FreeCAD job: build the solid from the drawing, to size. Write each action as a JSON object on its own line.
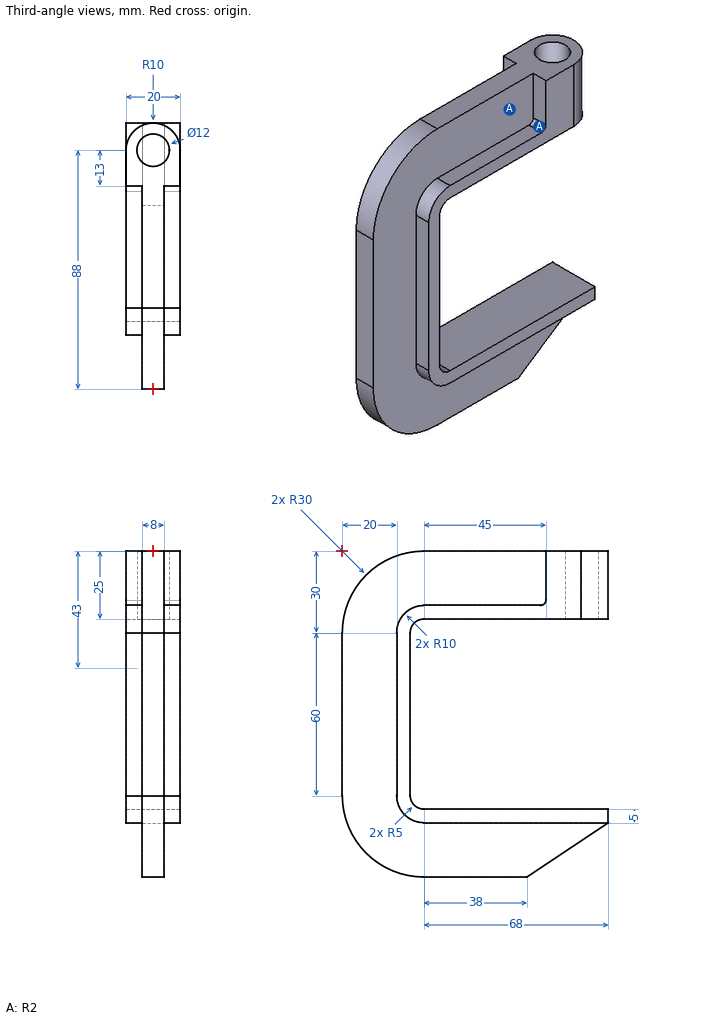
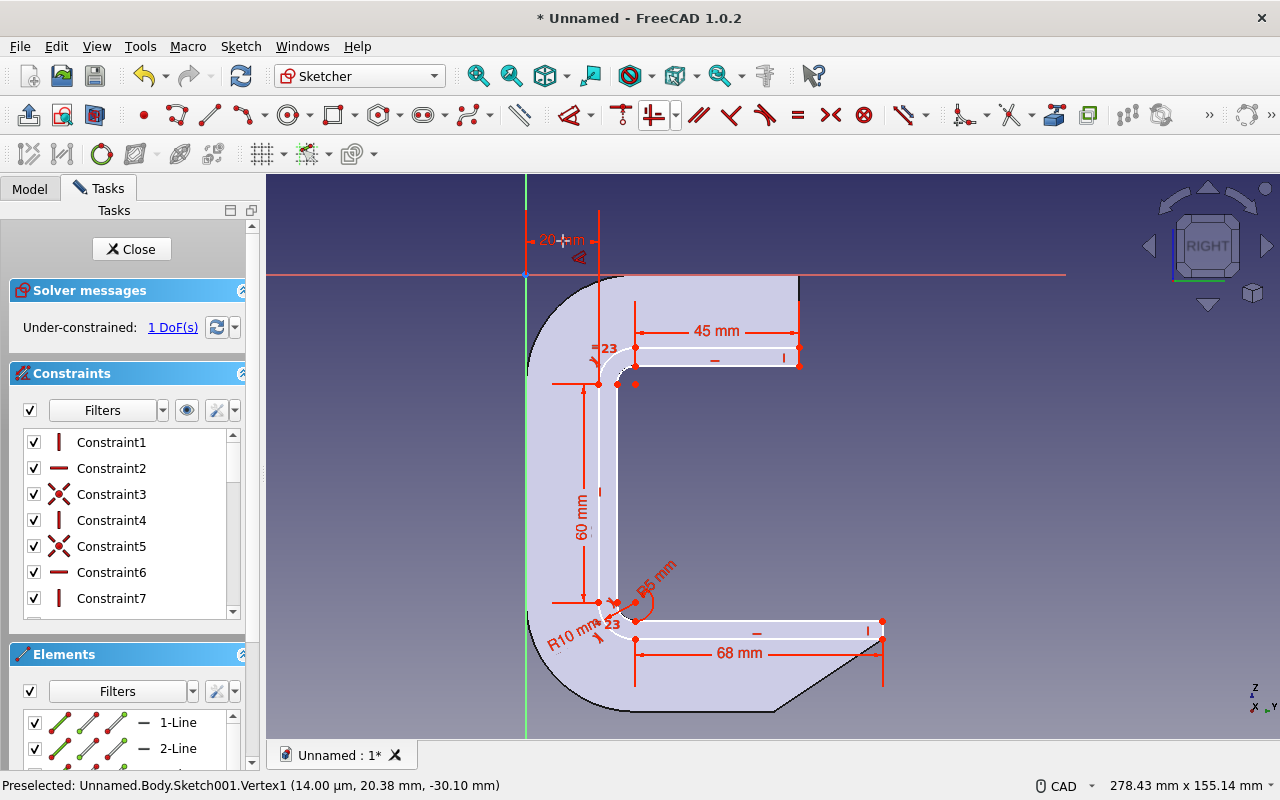
{"action": "left_click", "coordinate": [599, 384]}
{"action": "left_click", "coordinate": [492, 330]}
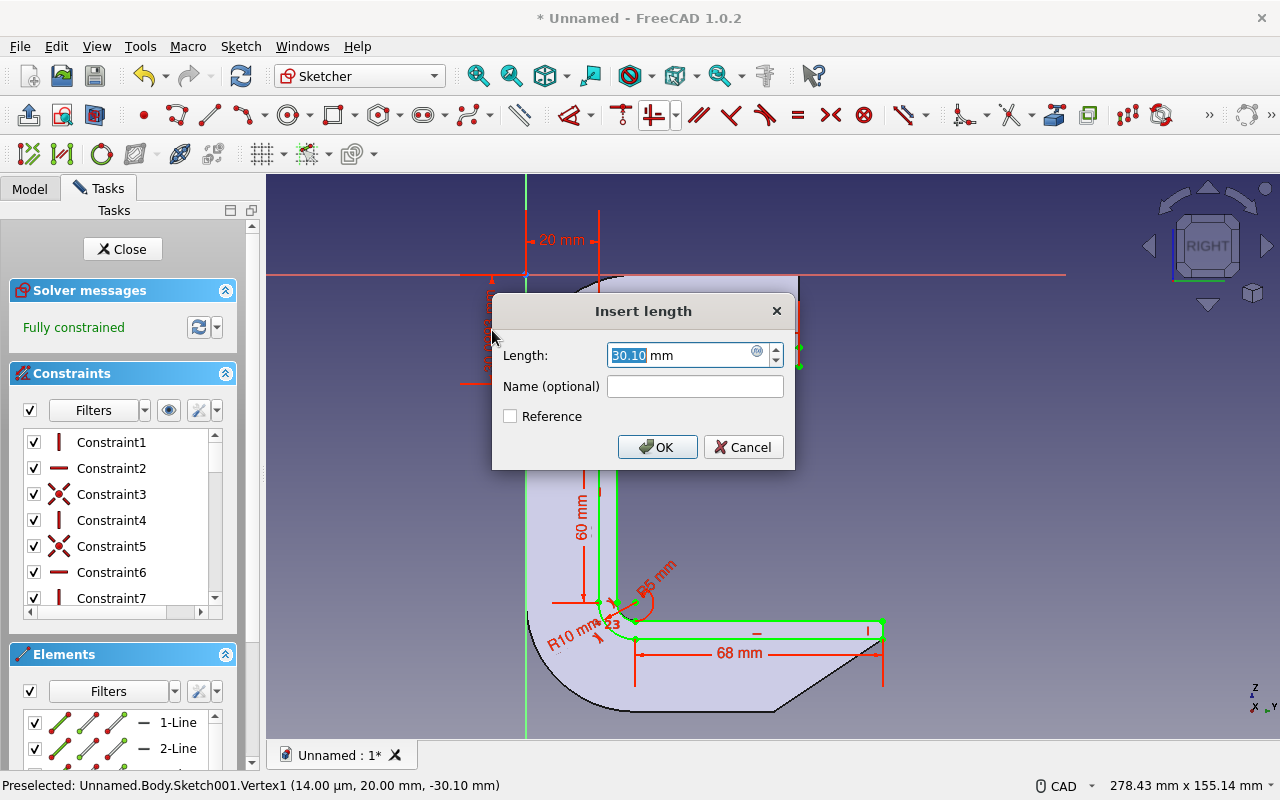
{"action": "type", "text": "30"}
{"action": "key", "text": "Return"}
{"action": "key", "text": "Escape"}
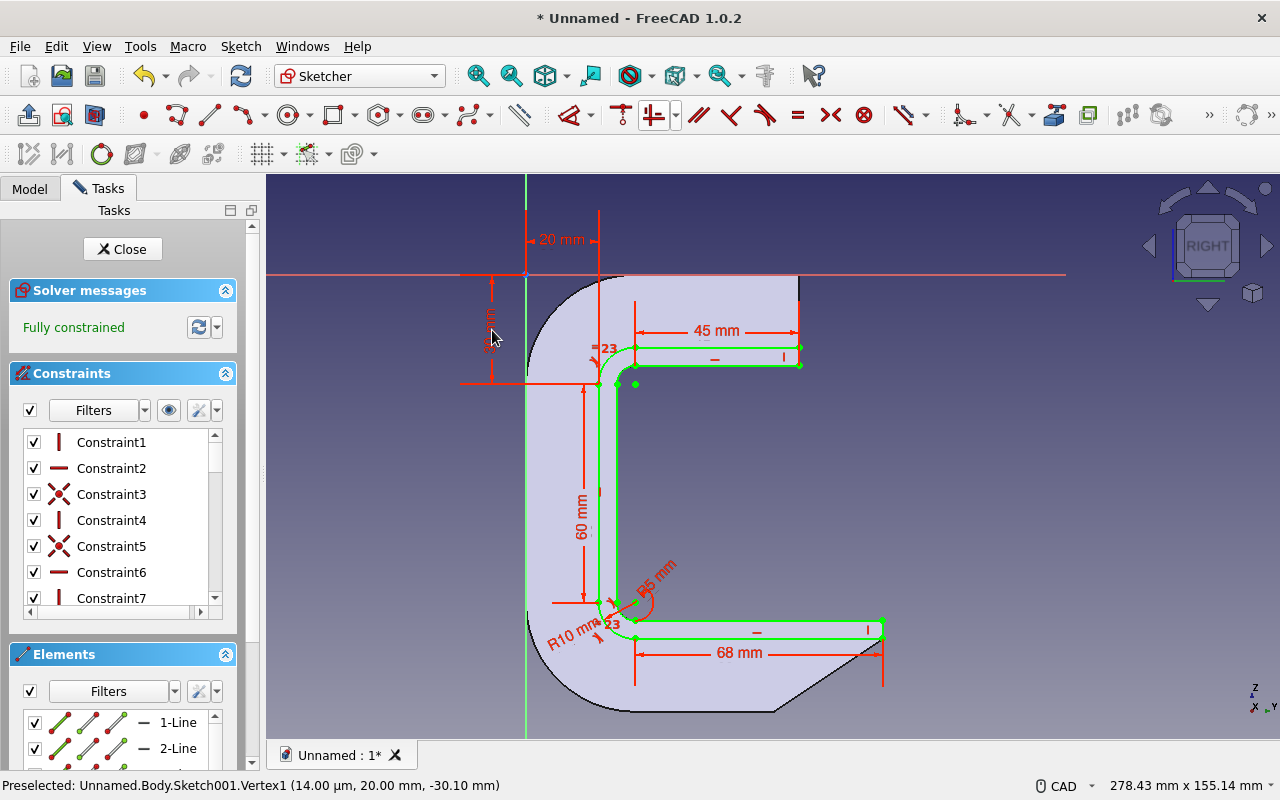
{"action": "left_click", "coordinate": [123, 249]}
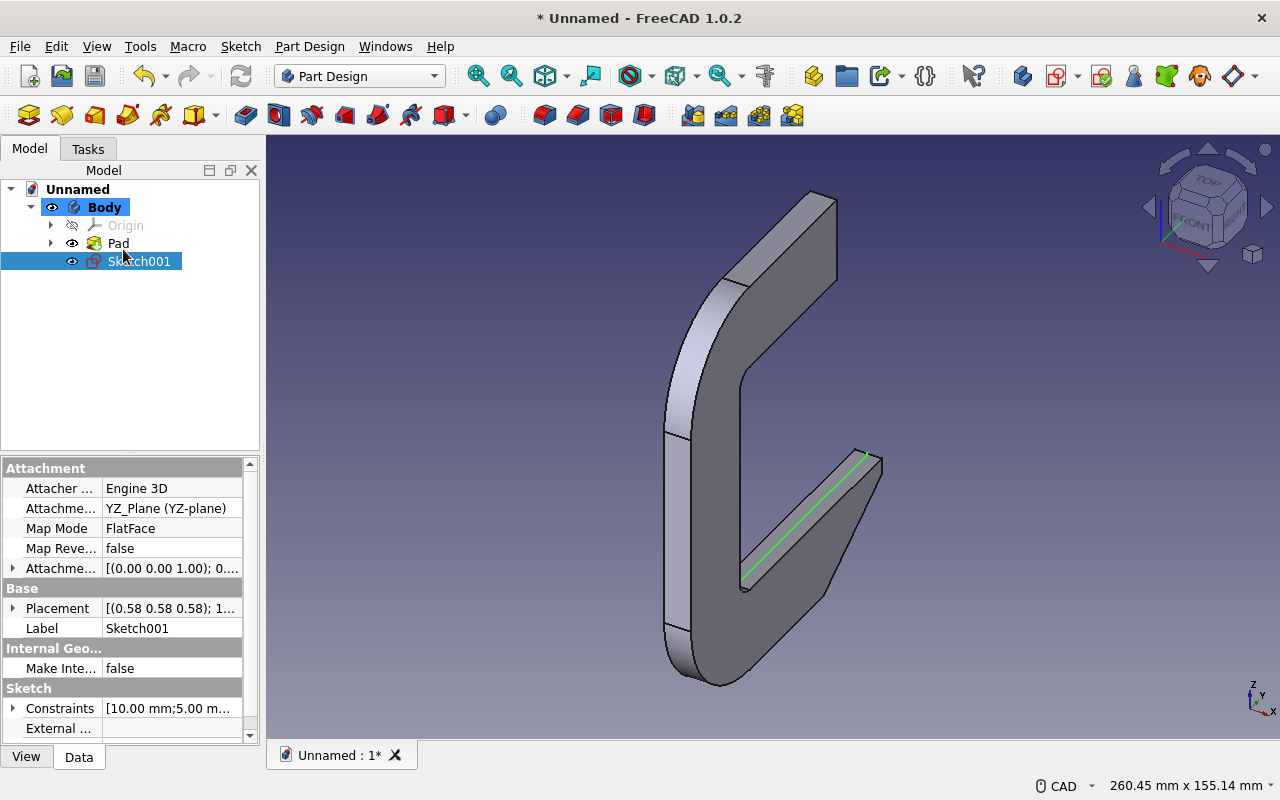
{"action": "left_click", "coordinate": [29, 116]}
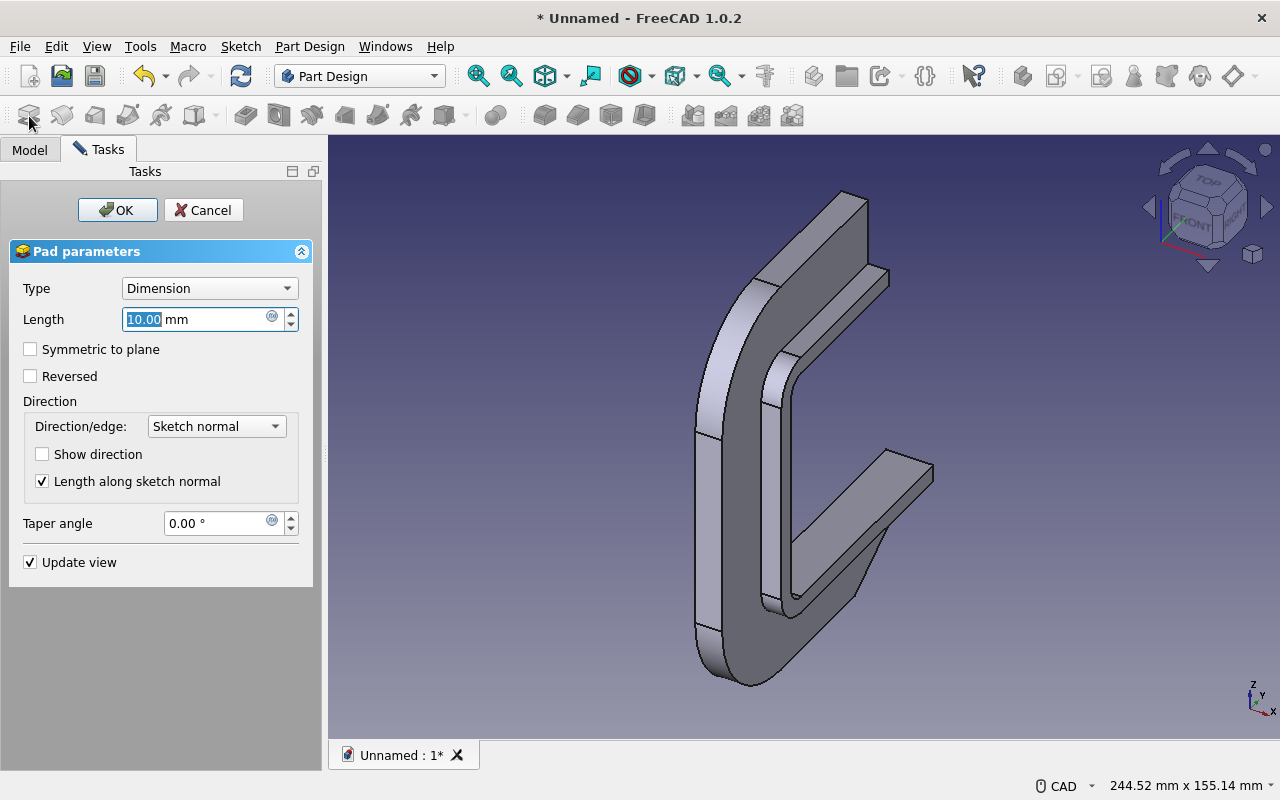
{"action": "type", "text": "20"}
{"action": "key", "text": "Tab"}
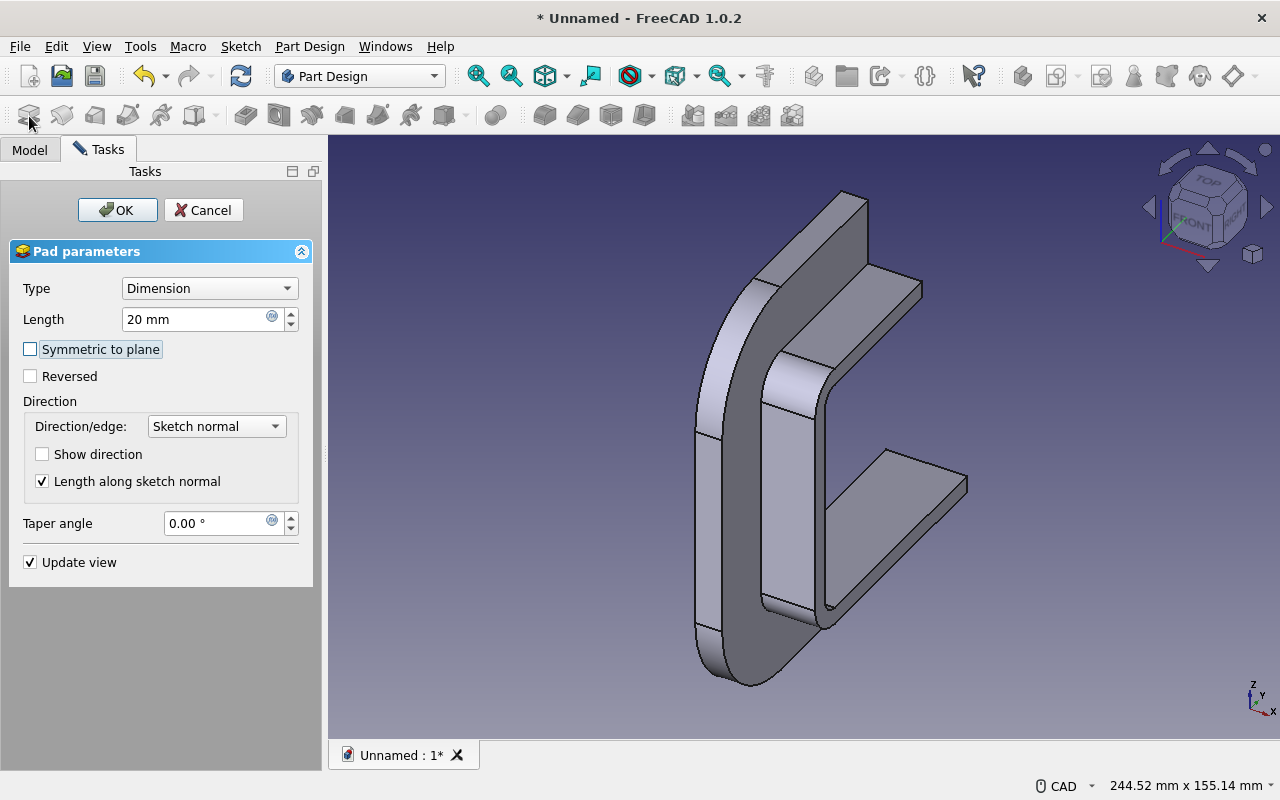
{"action": "left_click", "coordinate": [31, 349]}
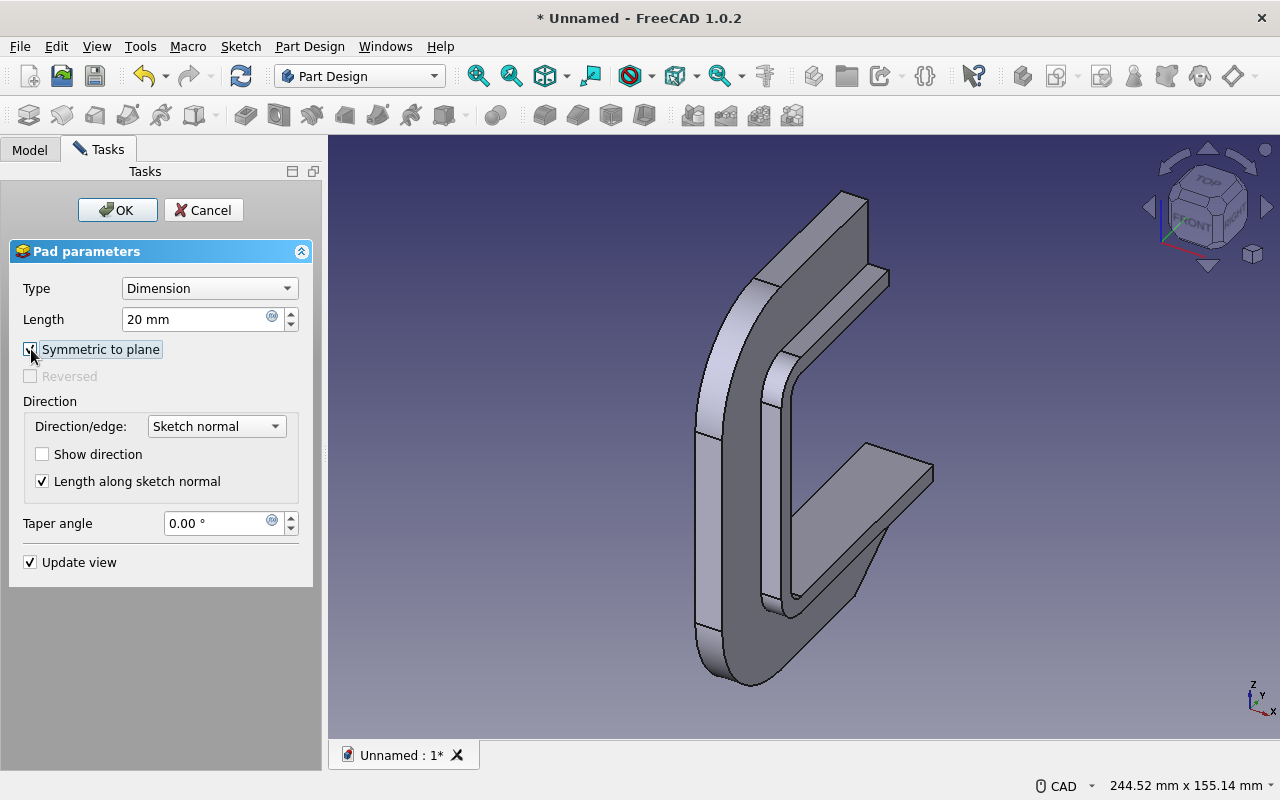
{"action": "left_click", "coordinate": [118, 210]}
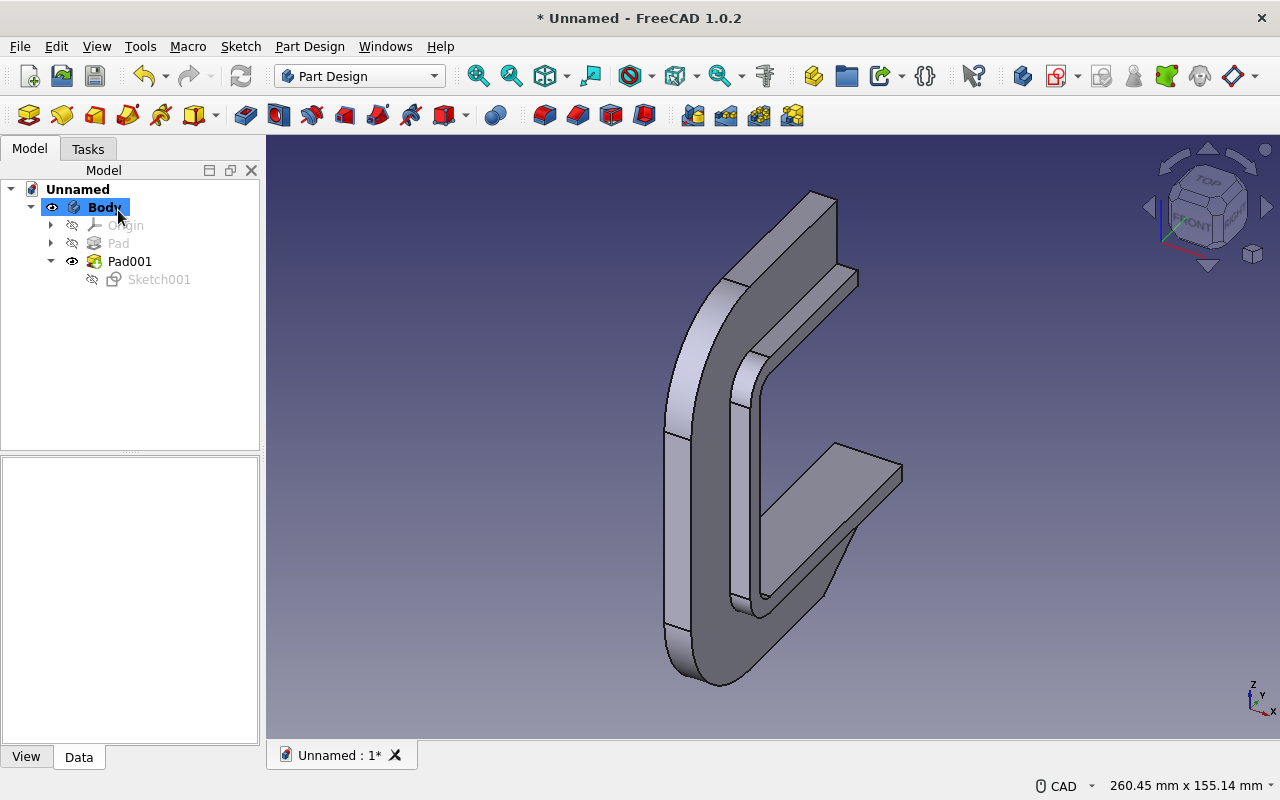
{"action": "left_click", "coordinate": [805, 213]}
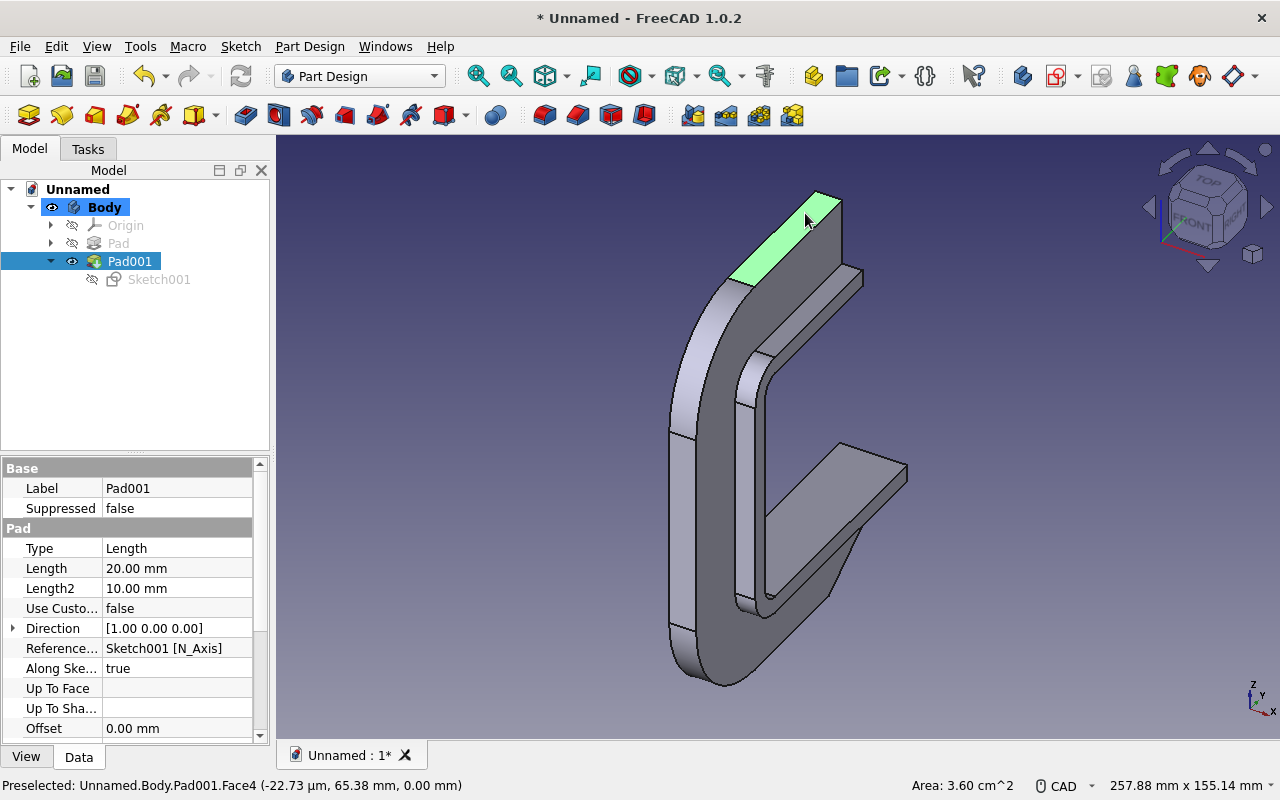
{"action": "left_click", "coordinate": [1056, 76]}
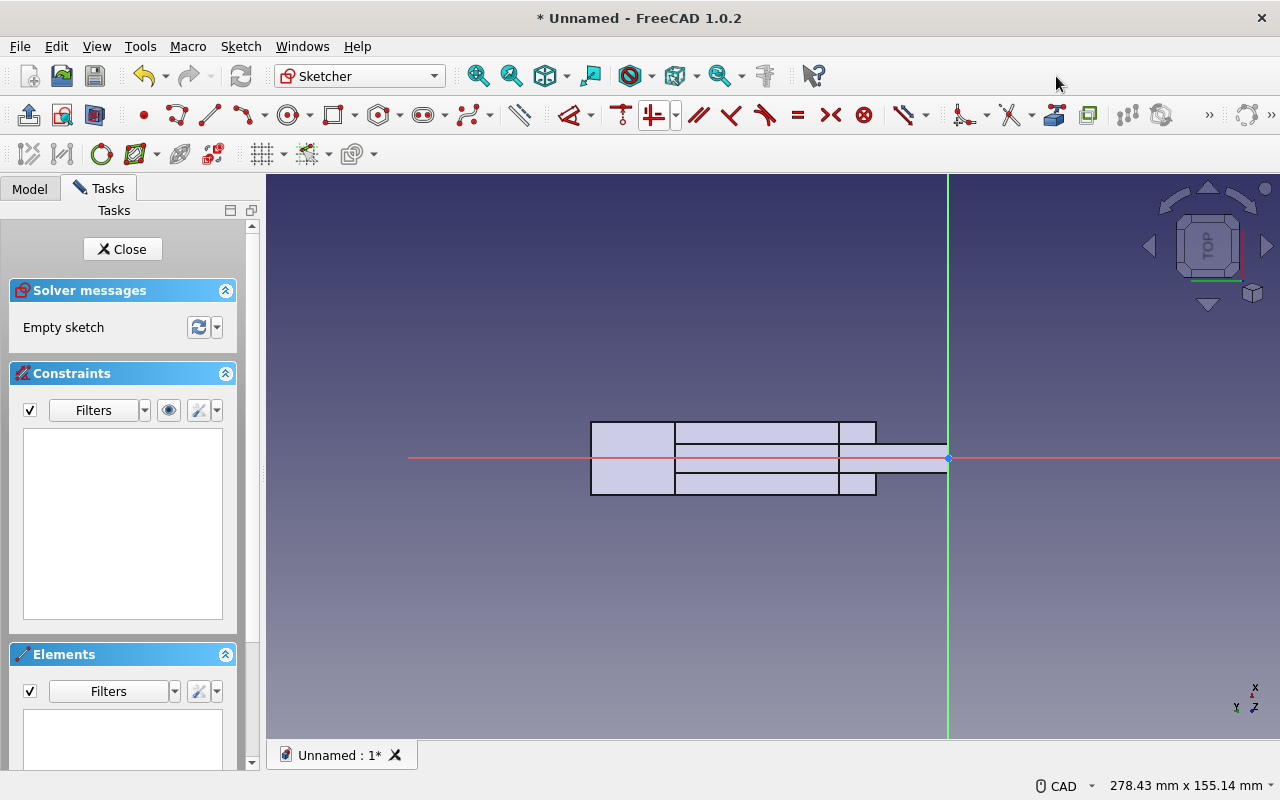
{"action": "scroll", "coordinate": [615, 458], "scroll_direction": "up", "scroll_amount": 8}